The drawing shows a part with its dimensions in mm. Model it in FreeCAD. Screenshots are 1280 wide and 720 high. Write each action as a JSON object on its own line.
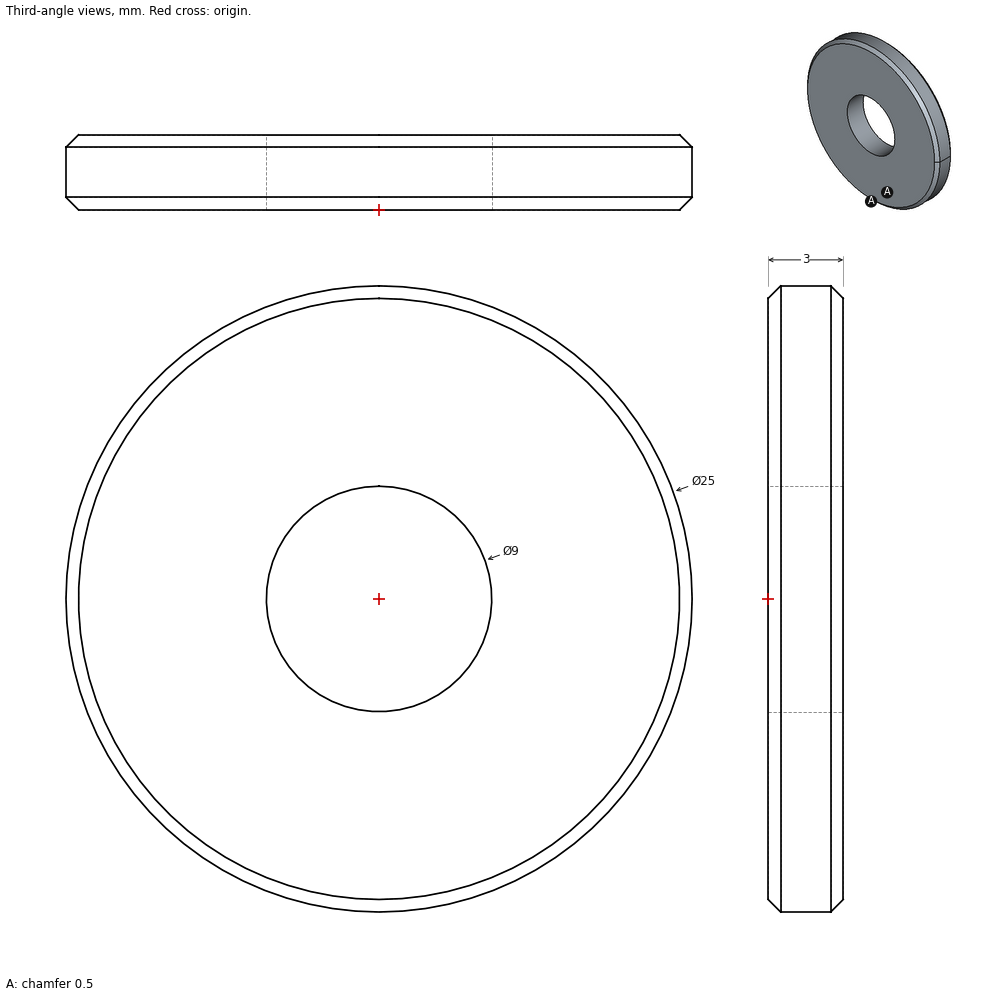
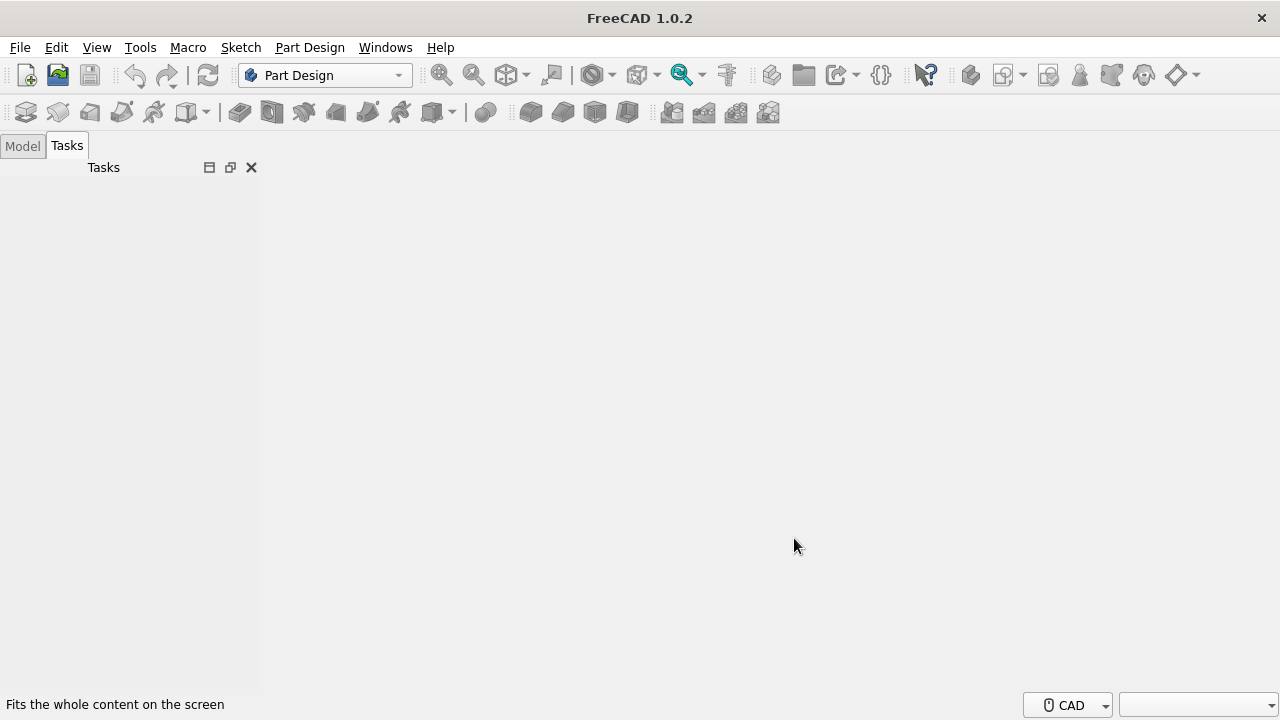
{"action": "left_click", "coordinate": [26, 76]}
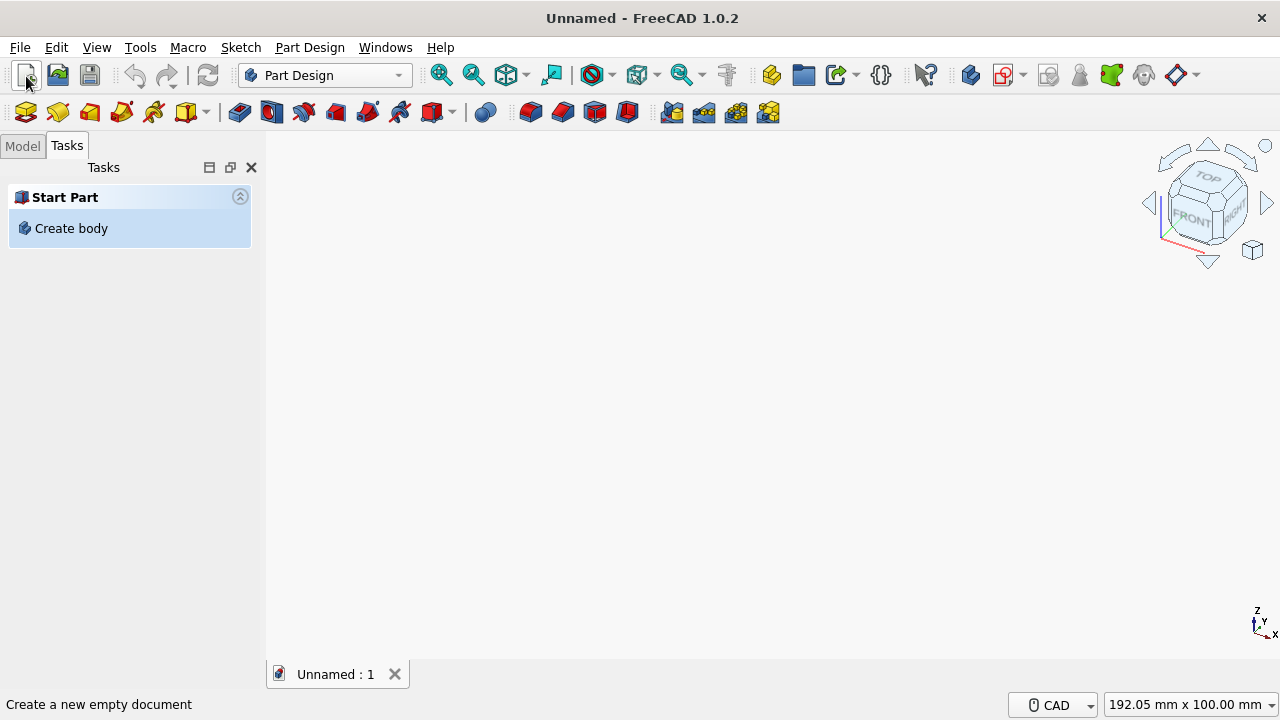
{"action": "left_click", "coordinate": [1004, 76]}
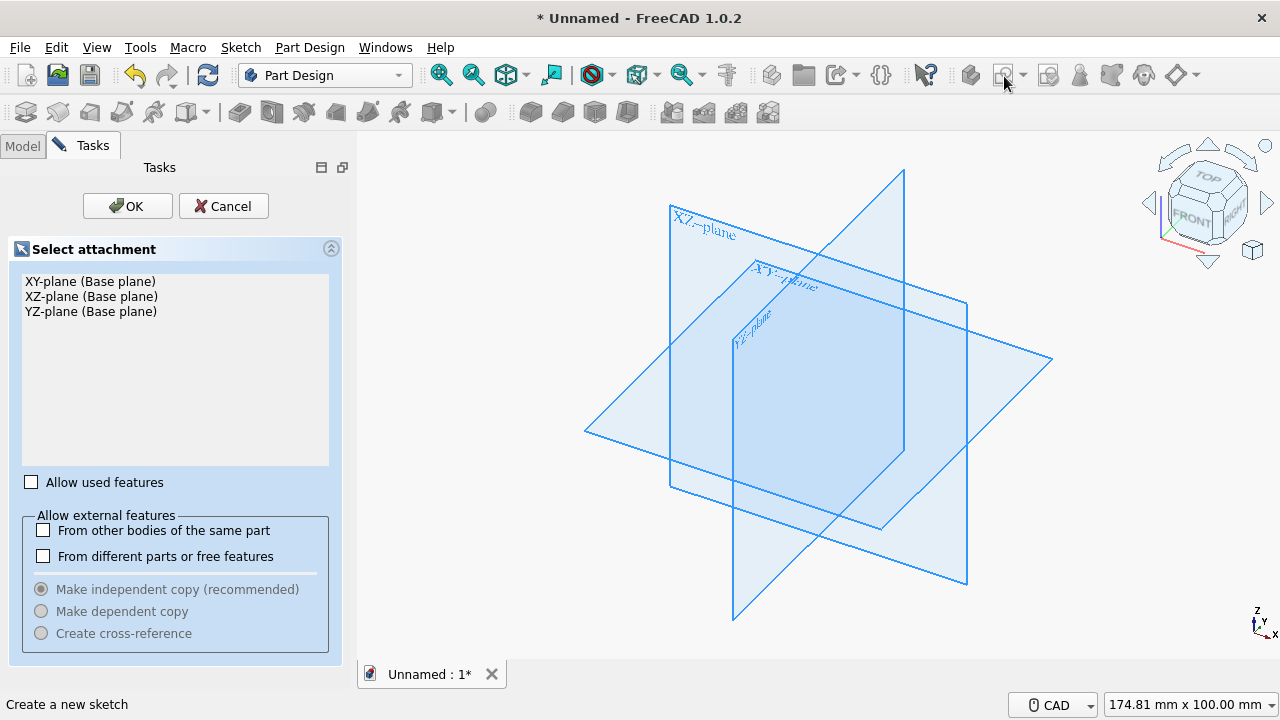
{"action": "left_click", "coordinate": [82, 296]}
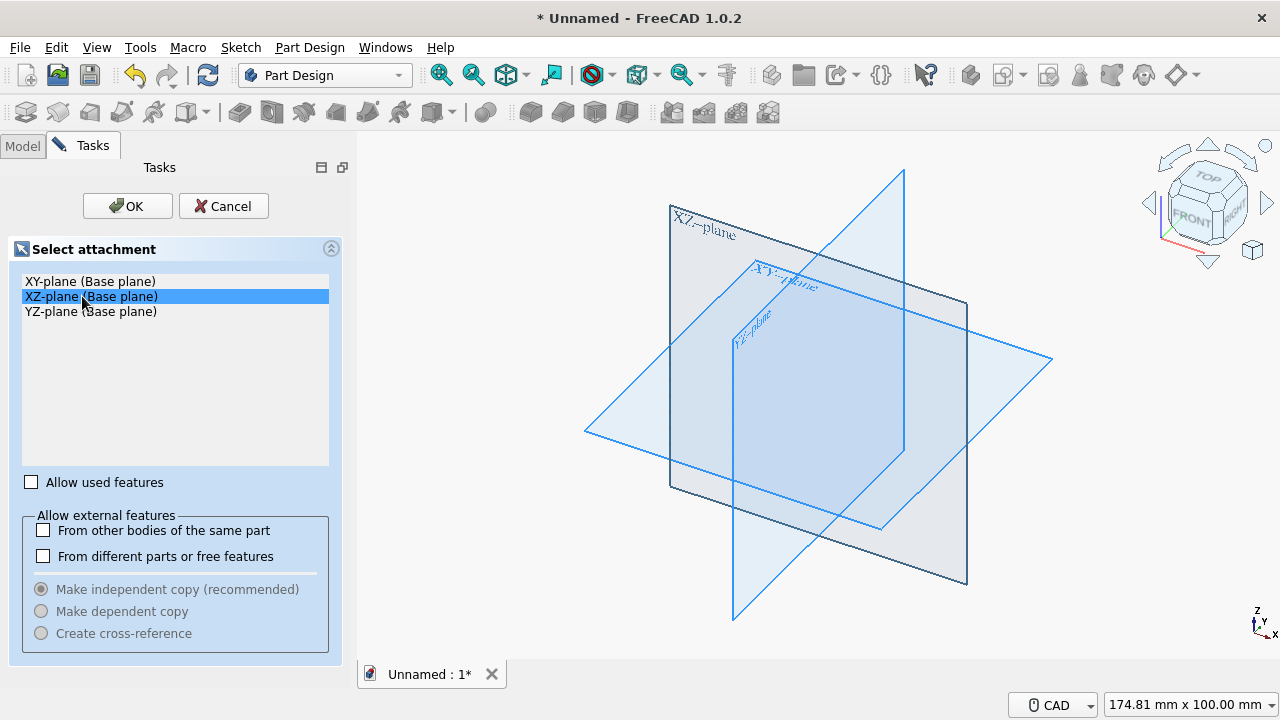
{"action": "left_click", "coordinate": [128, 206]}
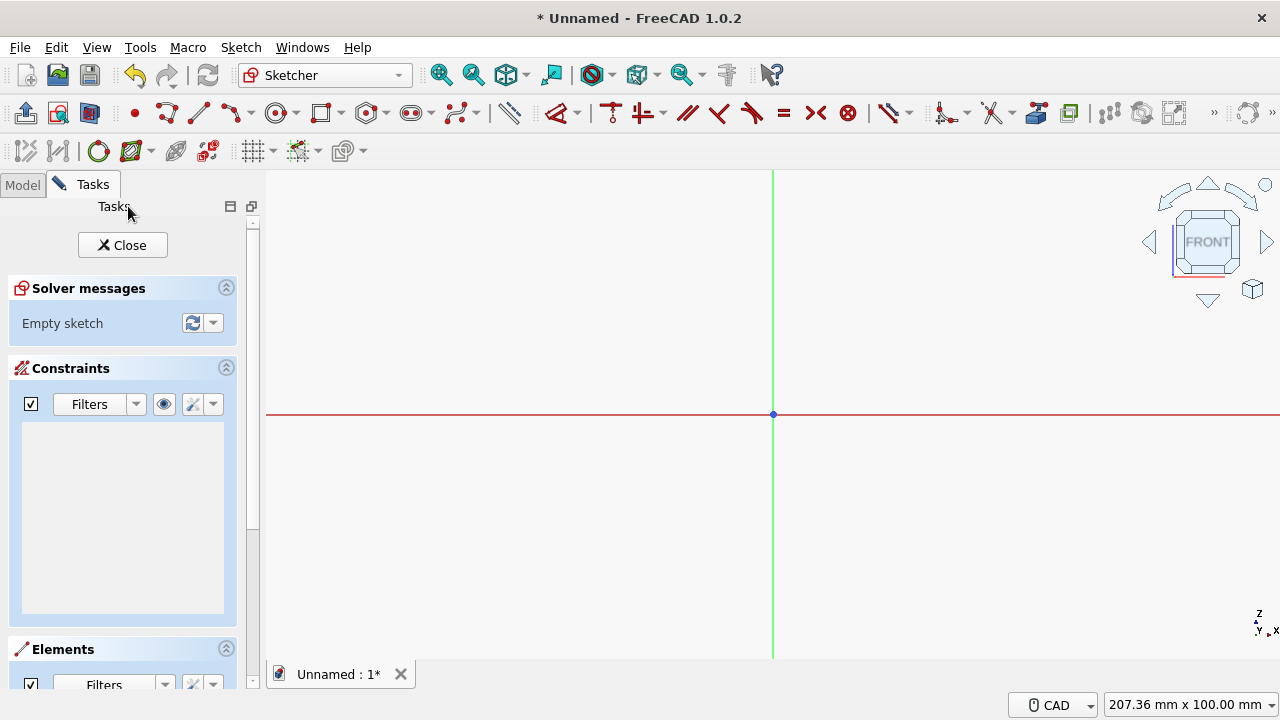
{"action": "scroll", "coordinate": [813, 415], "scroll_direction": "up", "scroll_amount": 5}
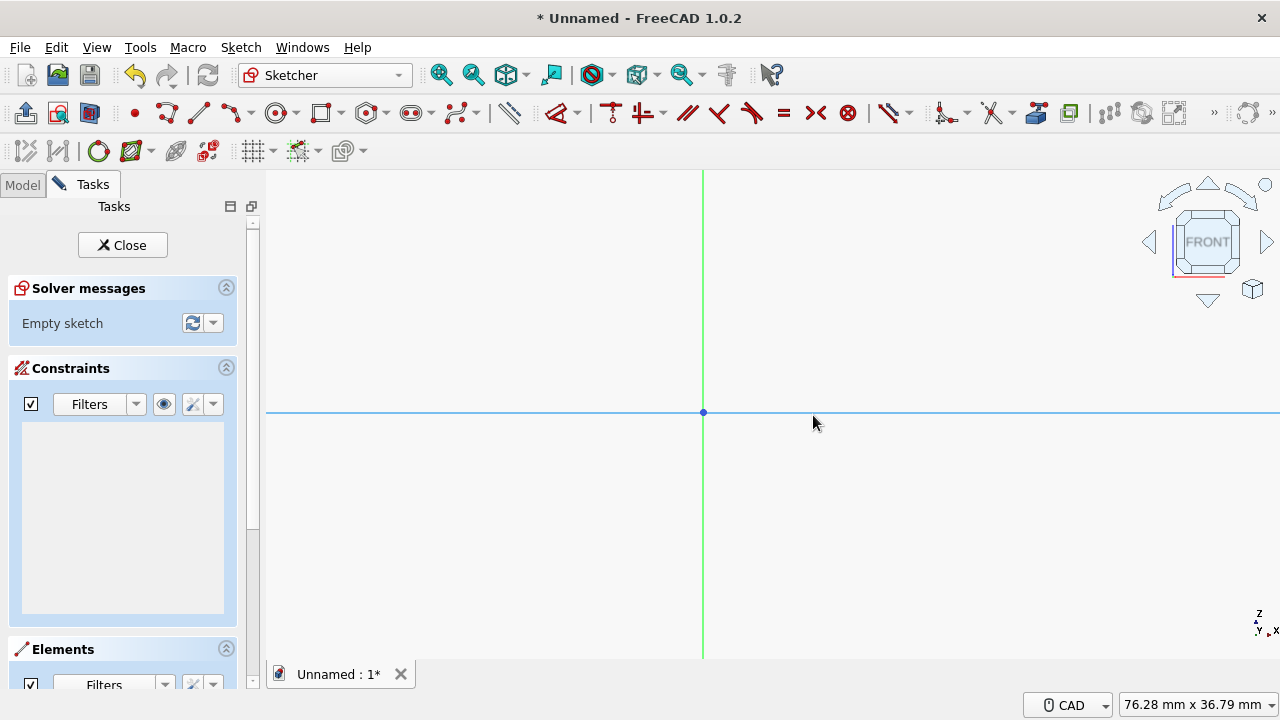
{"action": "left_click", "coordinate": [276, 114]}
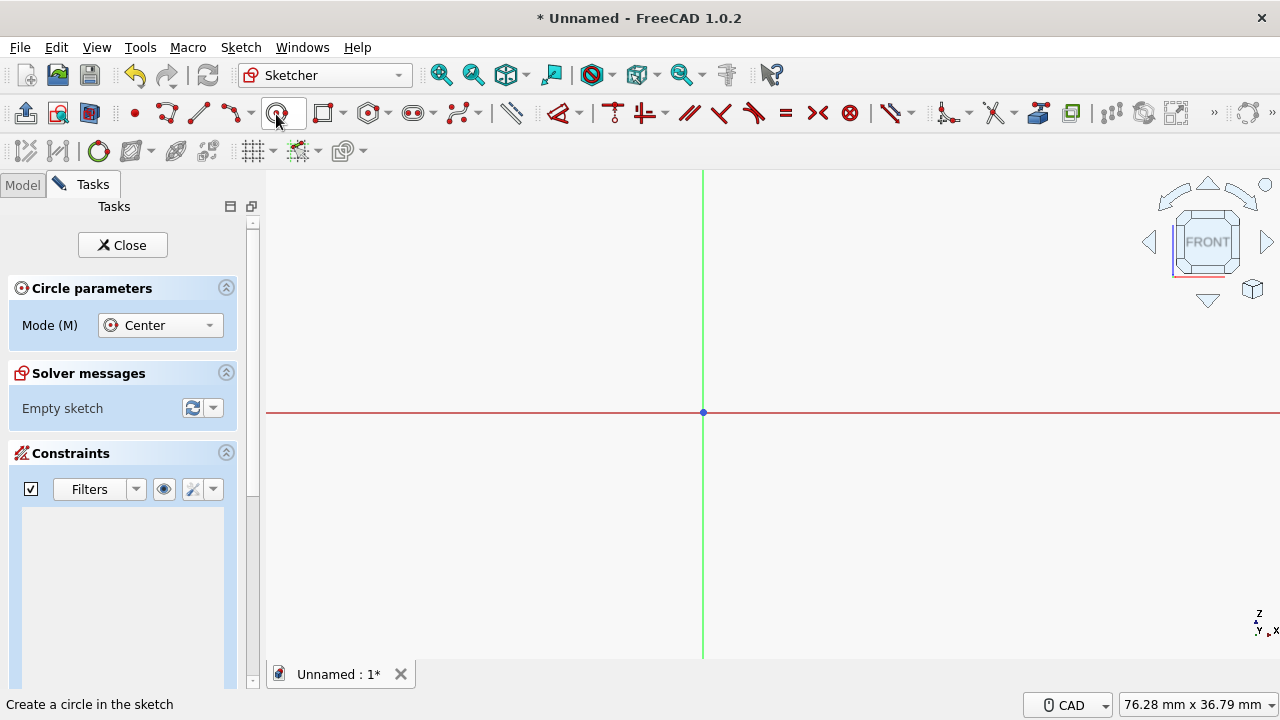
{"action": "left_click", "coordinate": [703, 413]}
{"action": "left_click", "coordinate": [821, 295]}
{"action": "key", "text": "Escape"}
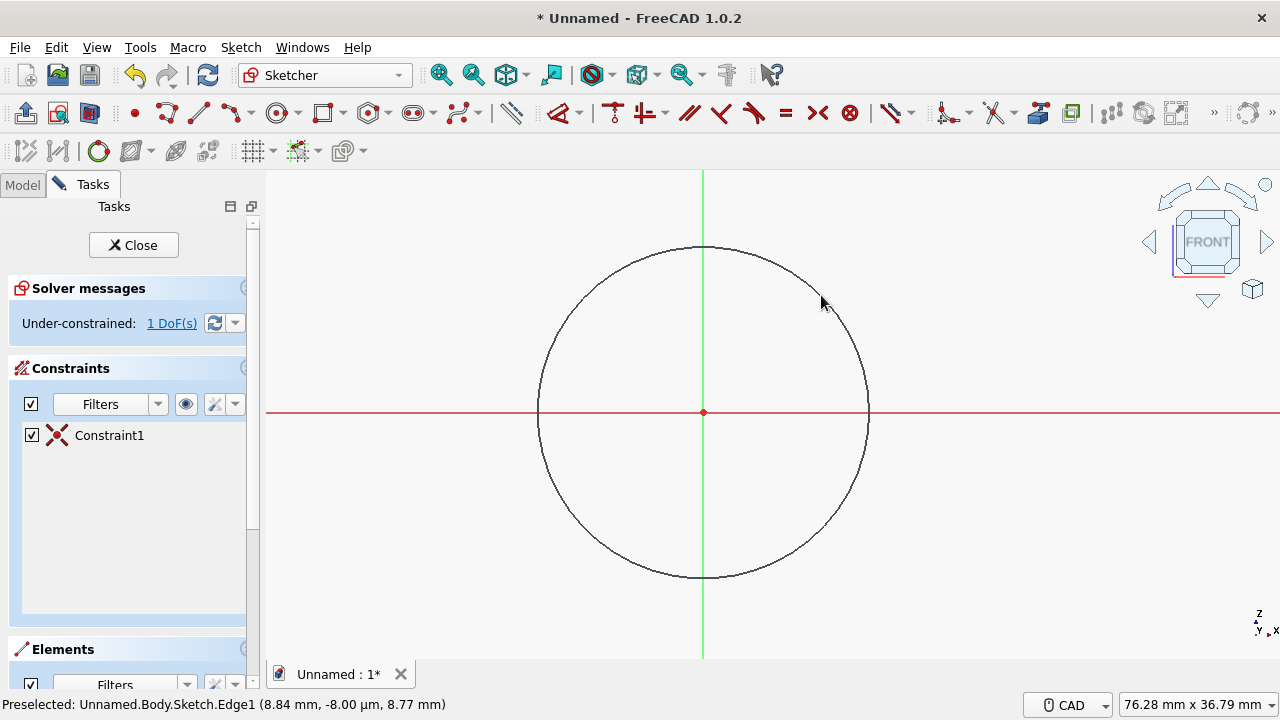
{"action": "left_click", "coordinate": [558, 114]}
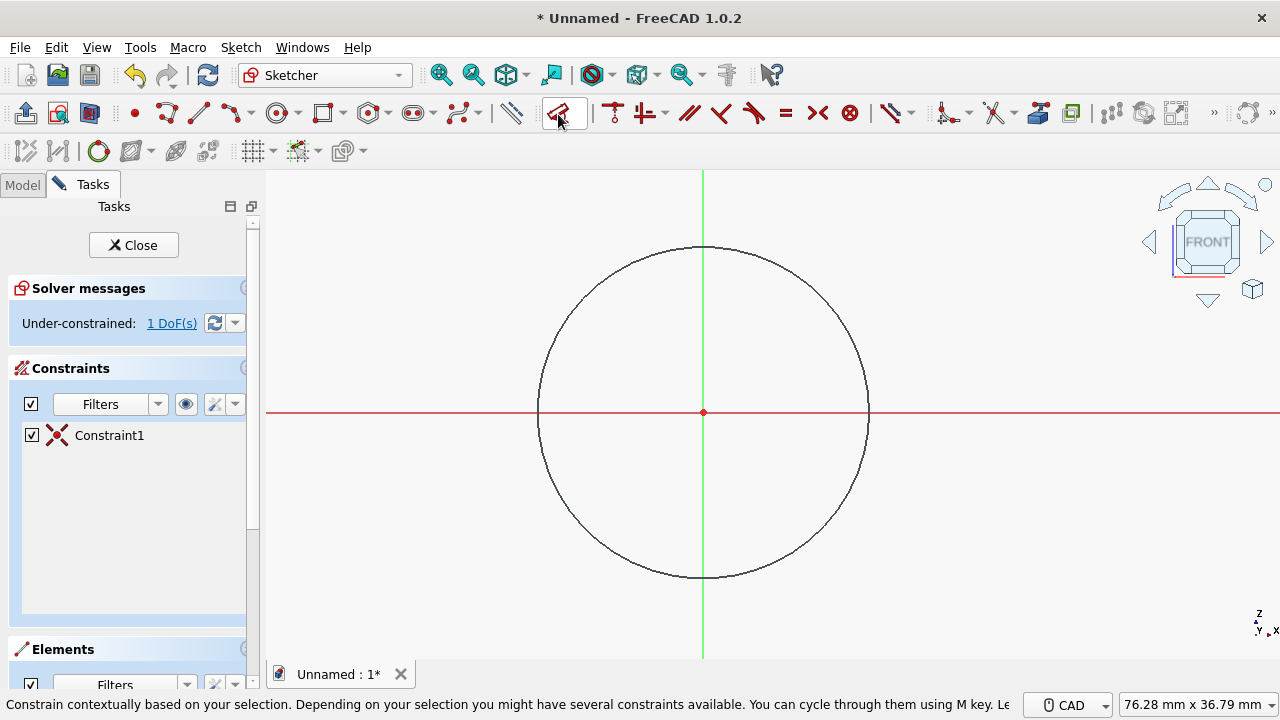
{"action": "left_click", "coordinate": [820, 295]}
{"action": "left_click", "coordinate": [843, 272]}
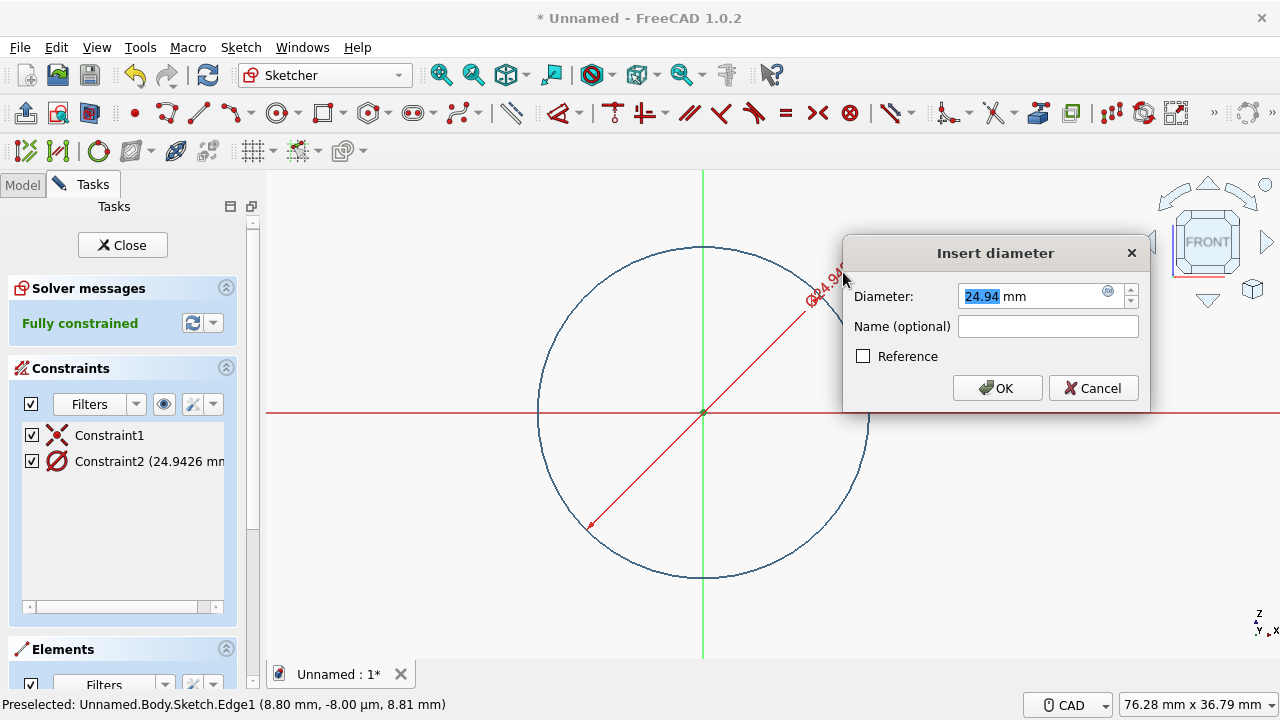
{"action": "type", "text": "25"}
{"action": "key", "text": "Return"}
{"action": "key", "text": "Escape"}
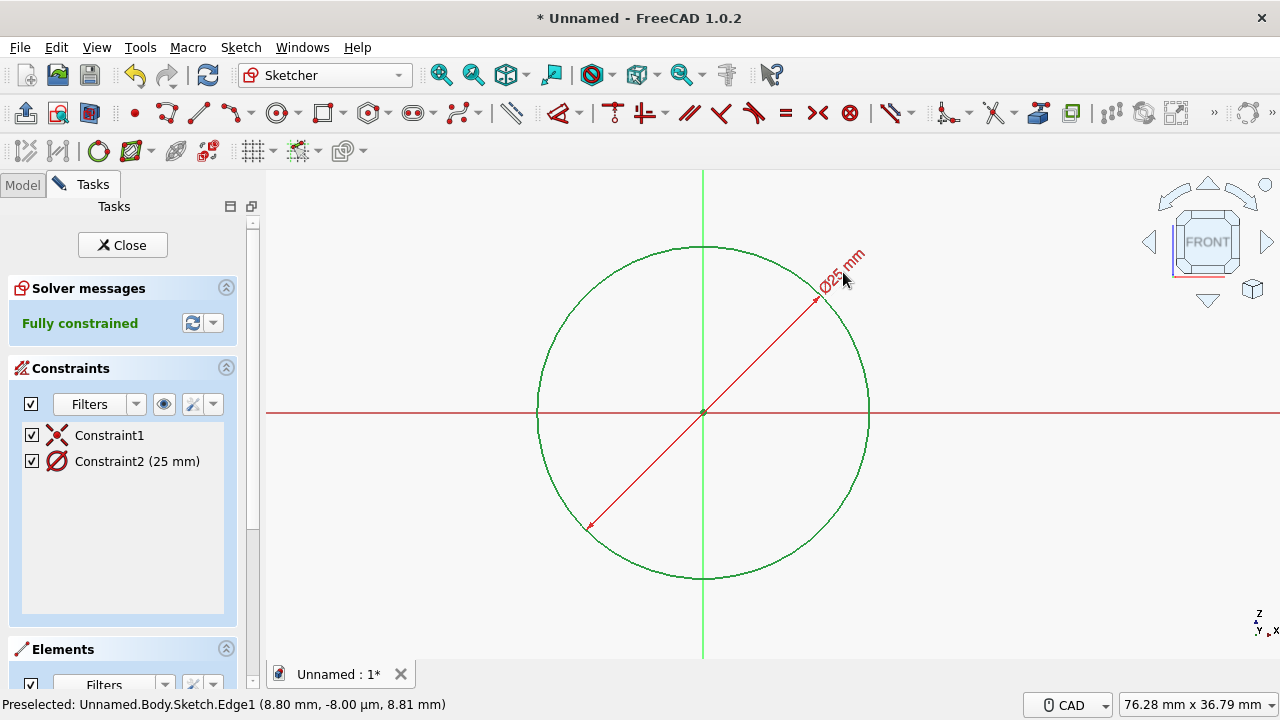
{"action": "left_click", "coordinate": [123, 245]}